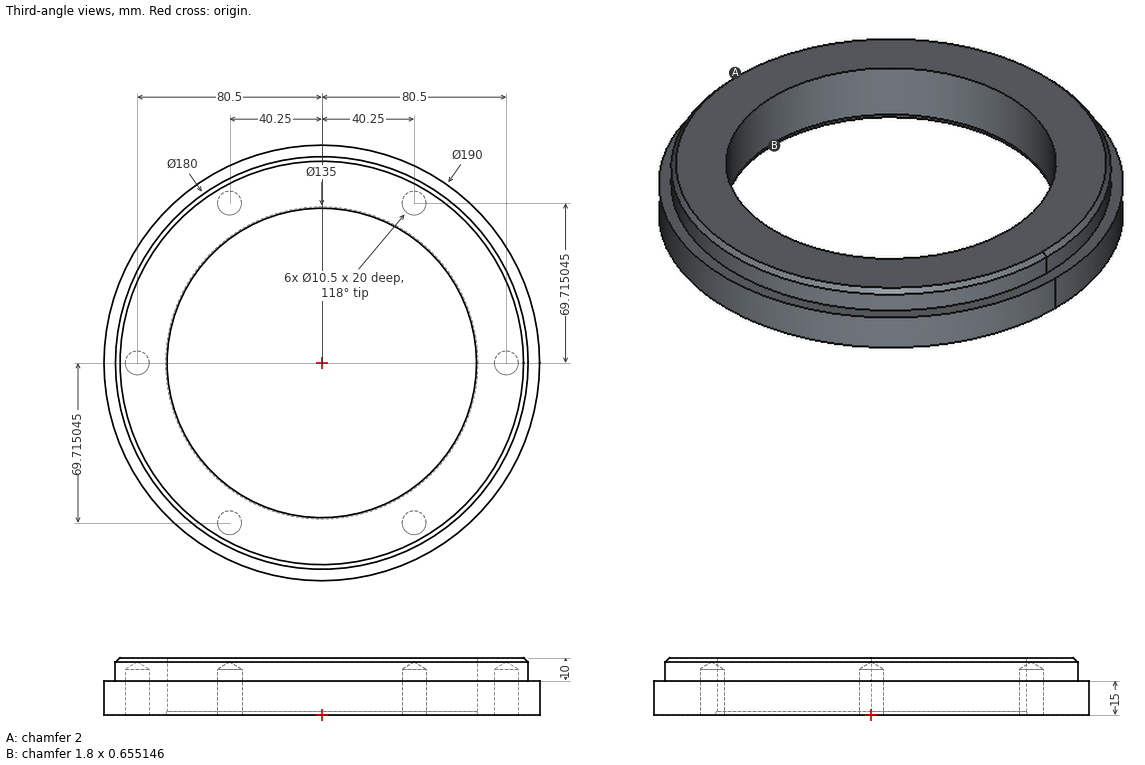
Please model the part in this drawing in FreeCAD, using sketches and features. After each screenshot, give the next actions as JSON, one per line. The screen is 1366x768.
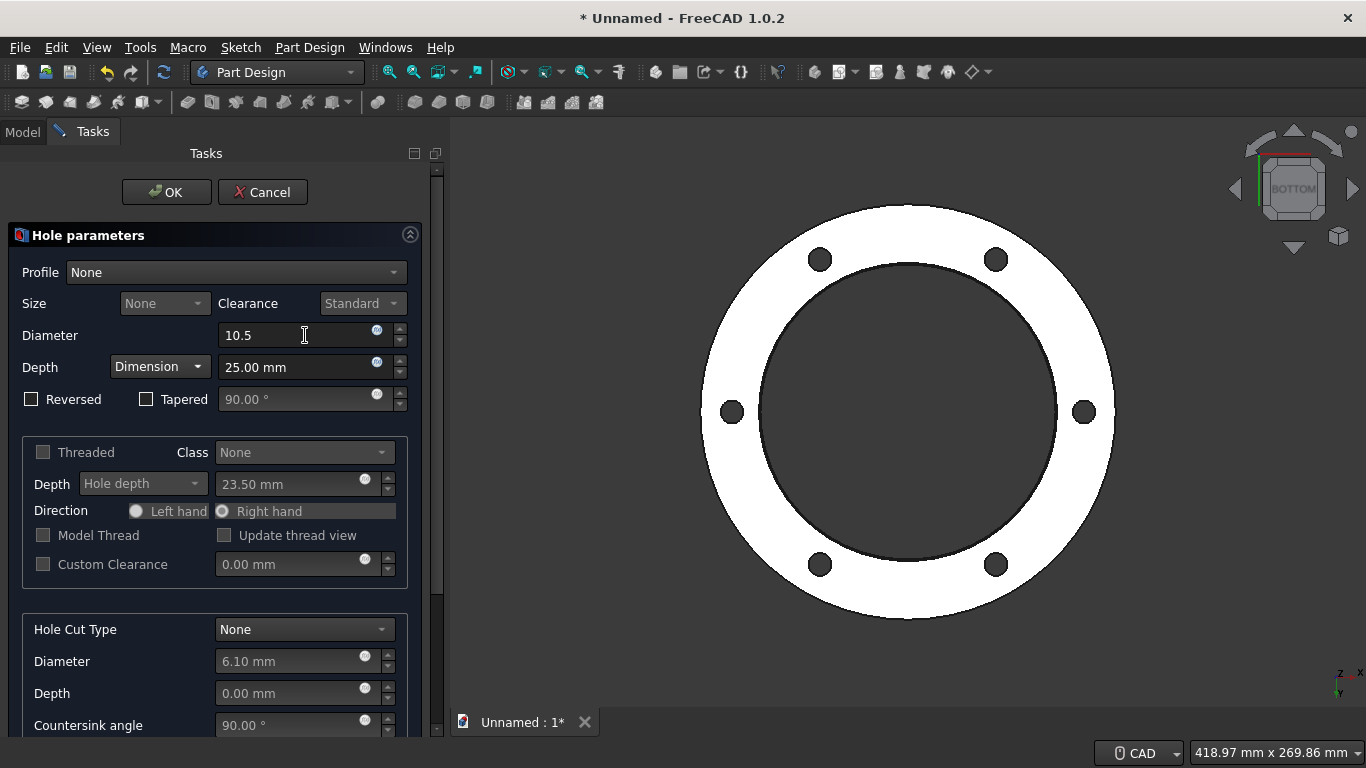
{"action": "triple_click", "coordinate": [305, 367]}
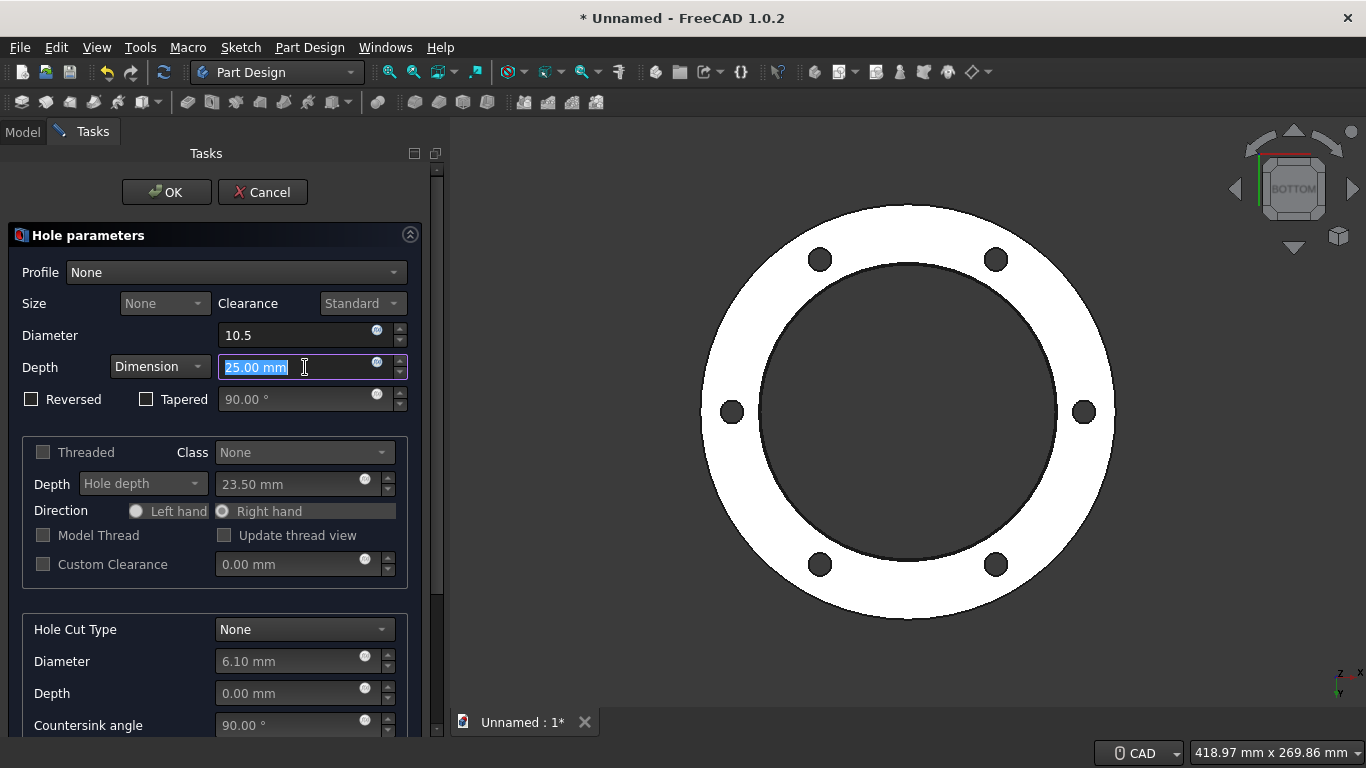
{"action": "type", "text": "20"}
{"action": "key", "text": "Tab"}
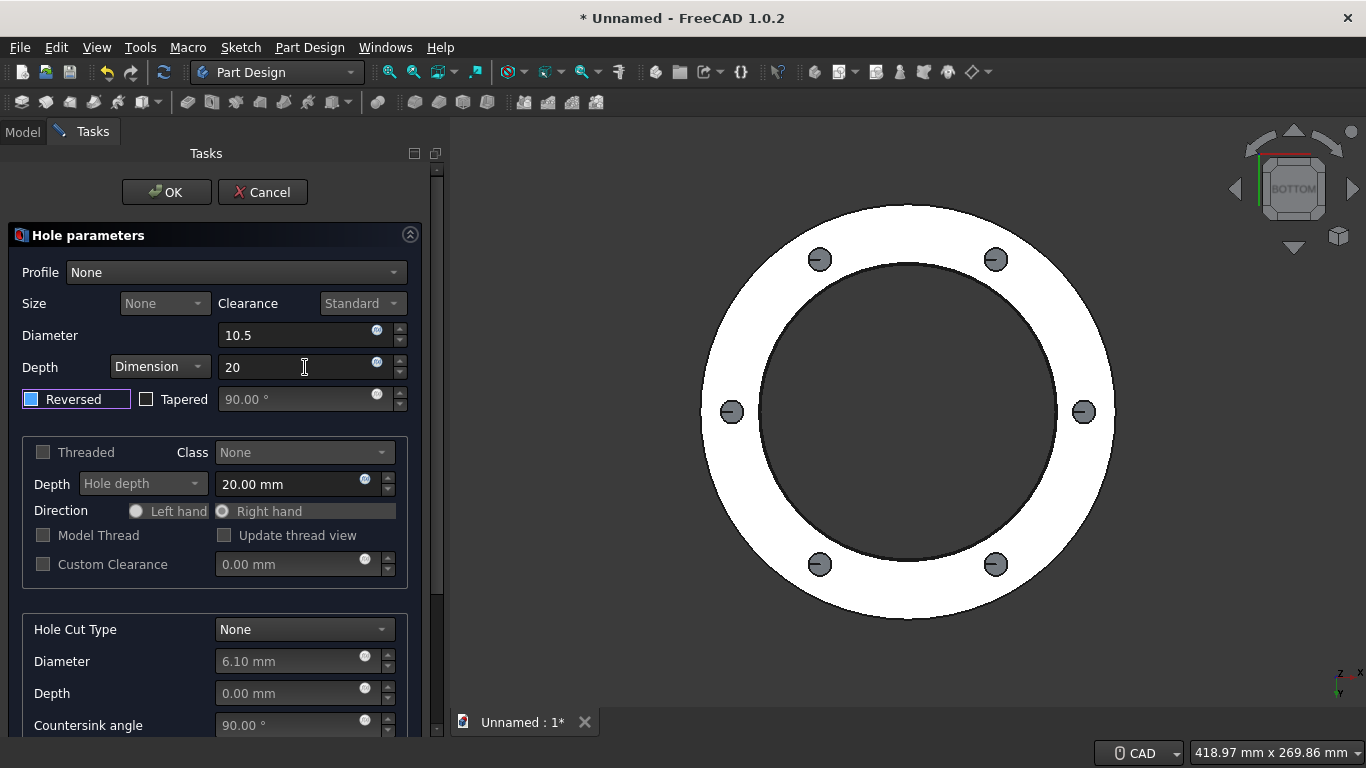
{"action": "left_click", "coordinate": [167, 192]}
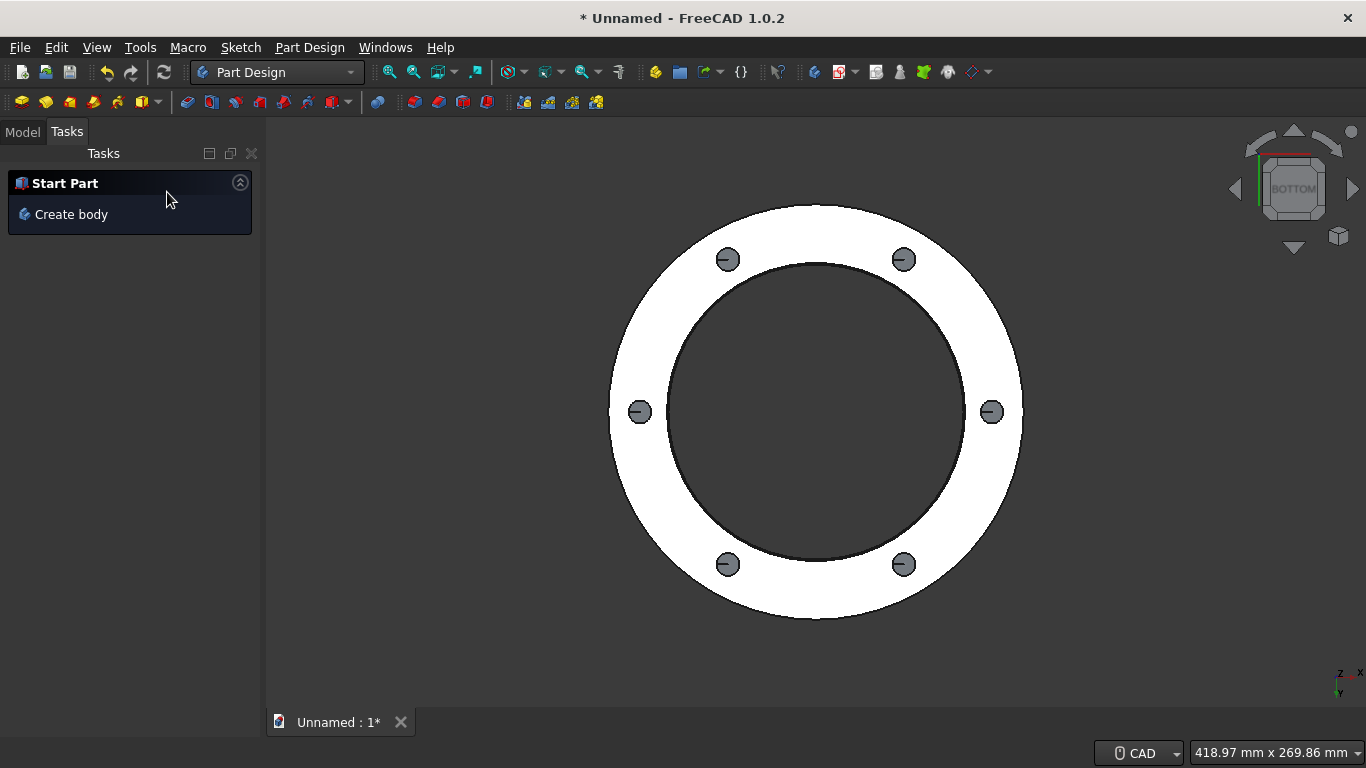
{"action": "key", "text": "0"}